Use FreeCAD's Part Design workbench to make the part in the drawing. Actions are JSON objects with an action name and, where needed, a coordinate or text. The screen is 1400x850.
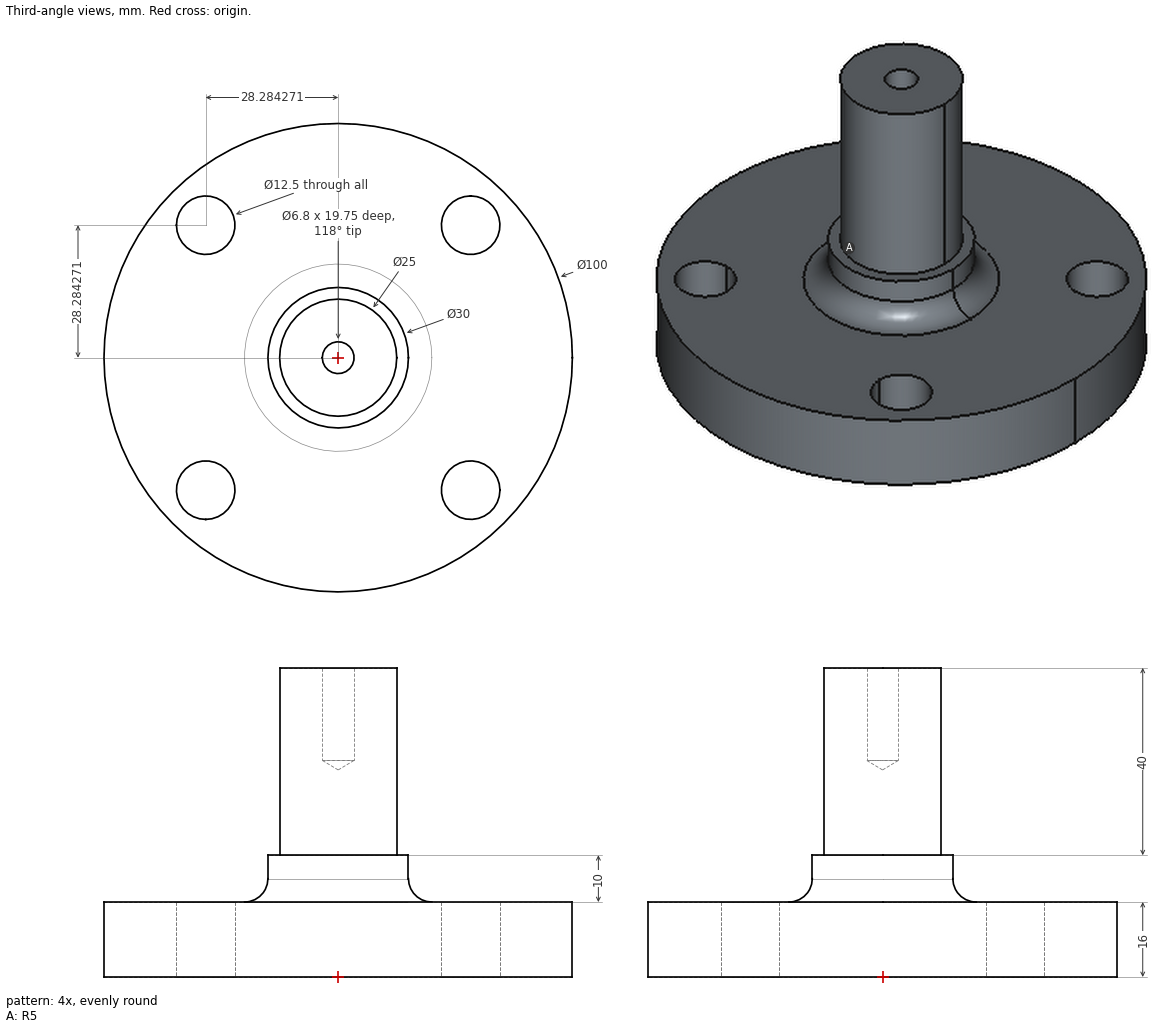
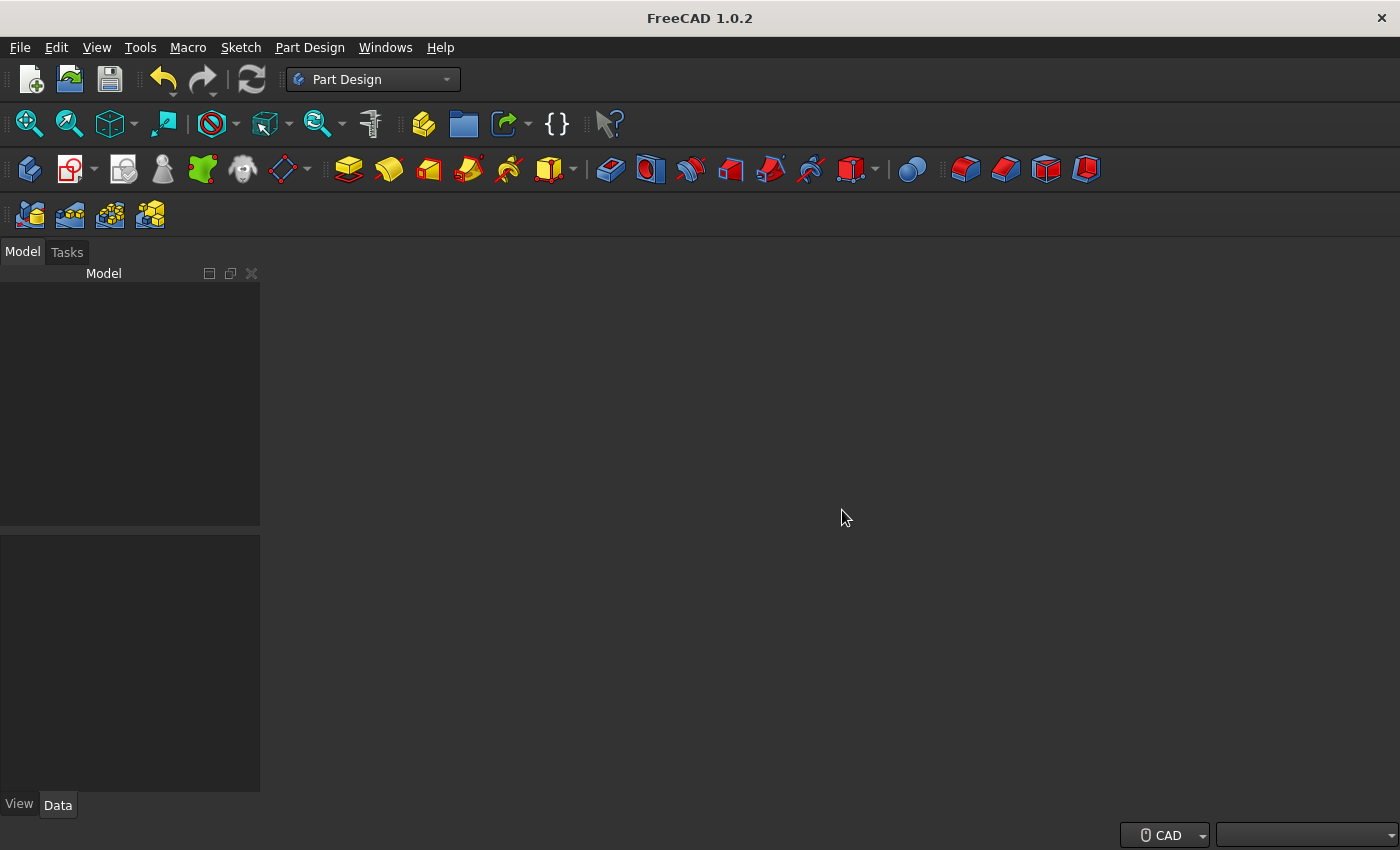
{"action": "key", "text": "ctrl+n"}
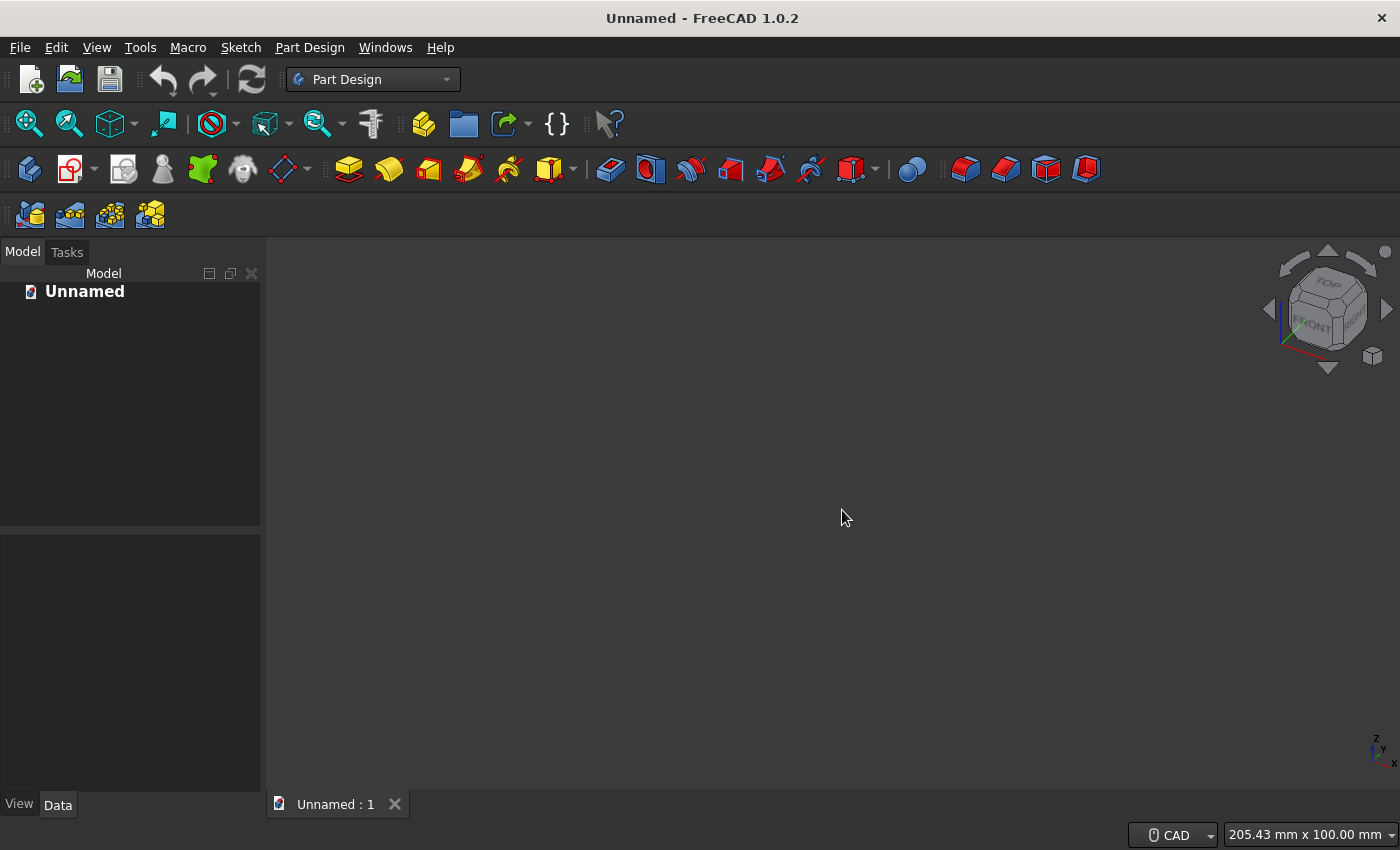
{"action": "left_click", "coordinate": [70, 170]}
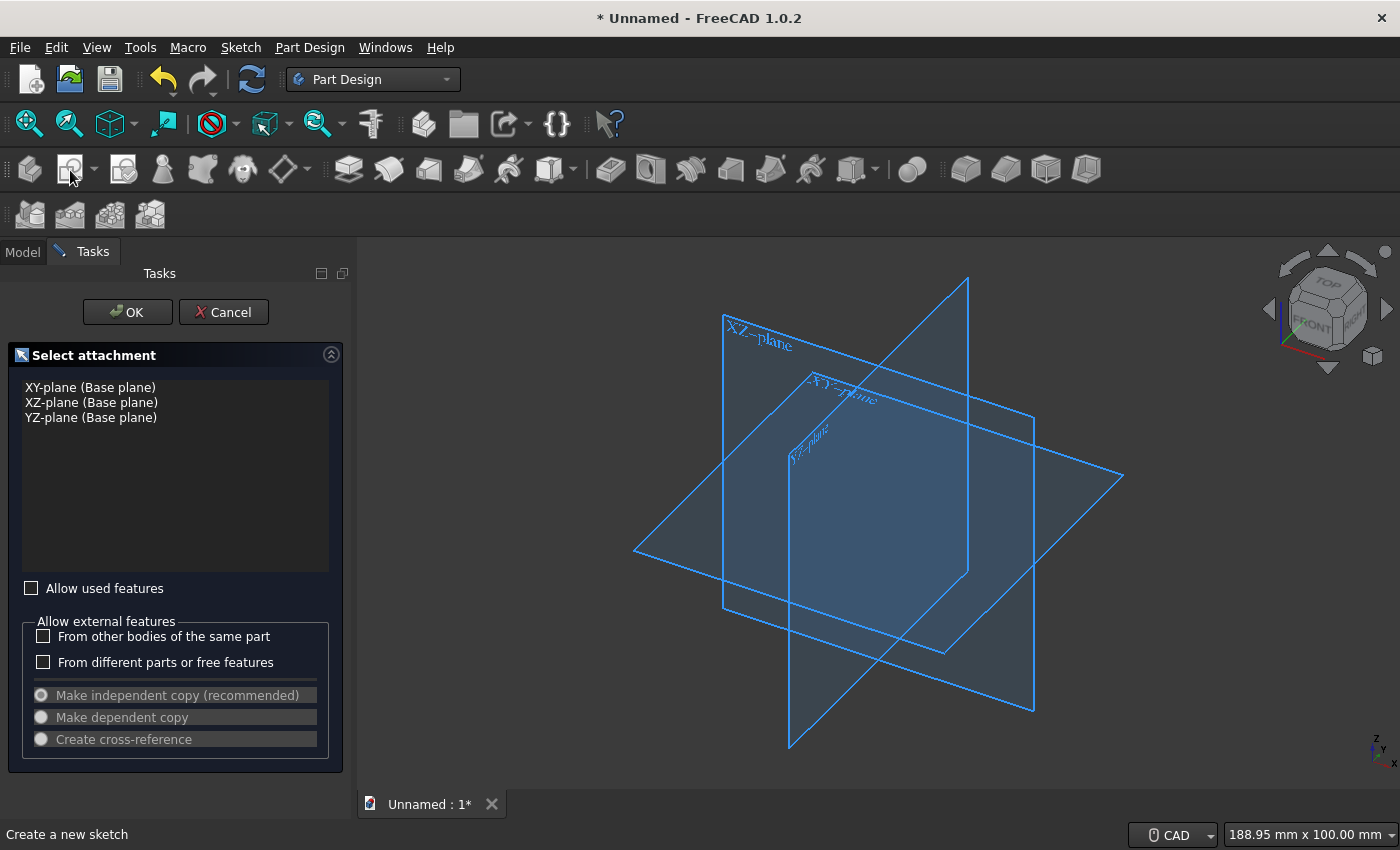
{"action": "left_click", "coordinate": [82, 388]}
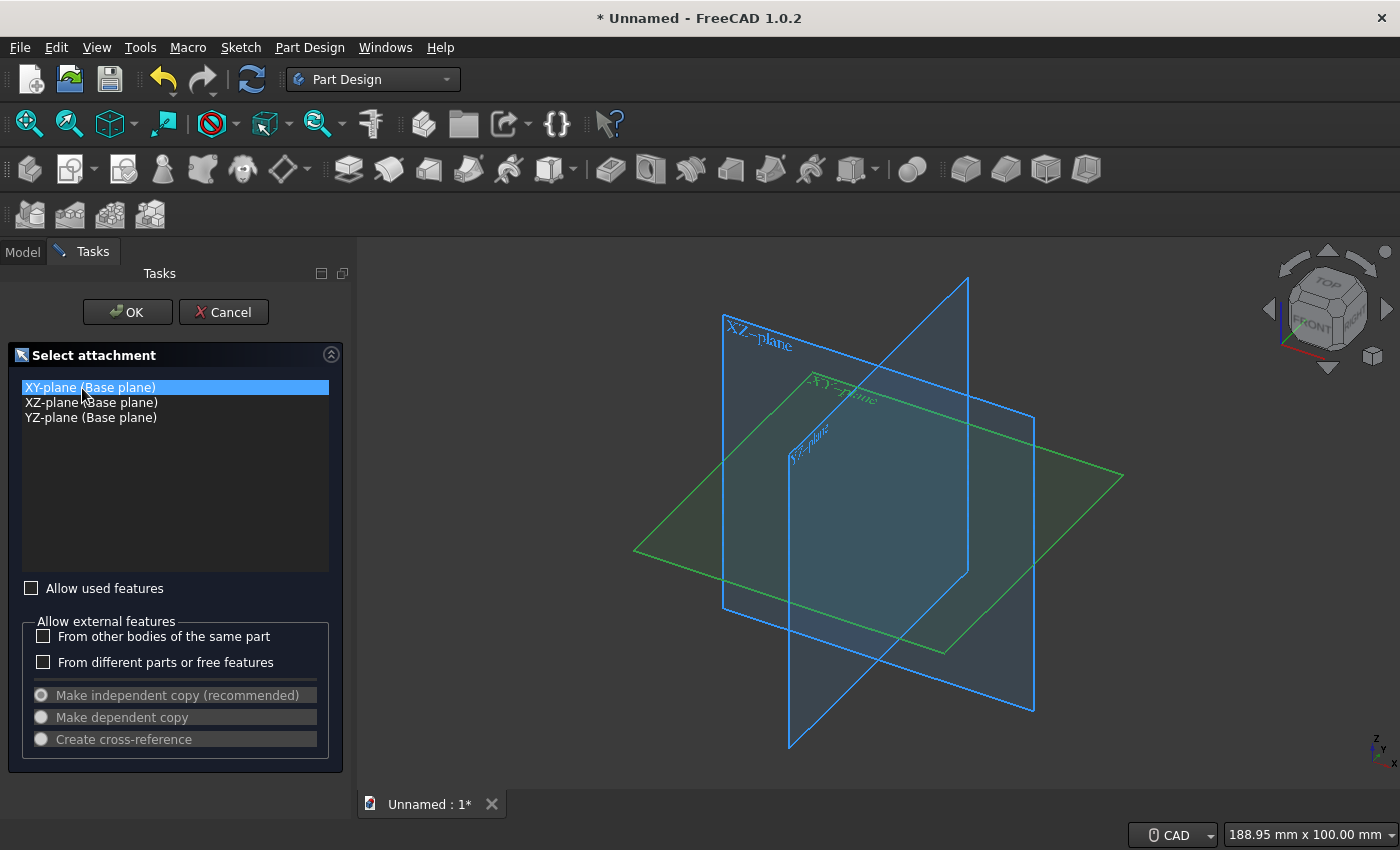
{"action": "left_click", "coordinate": [128, 312]}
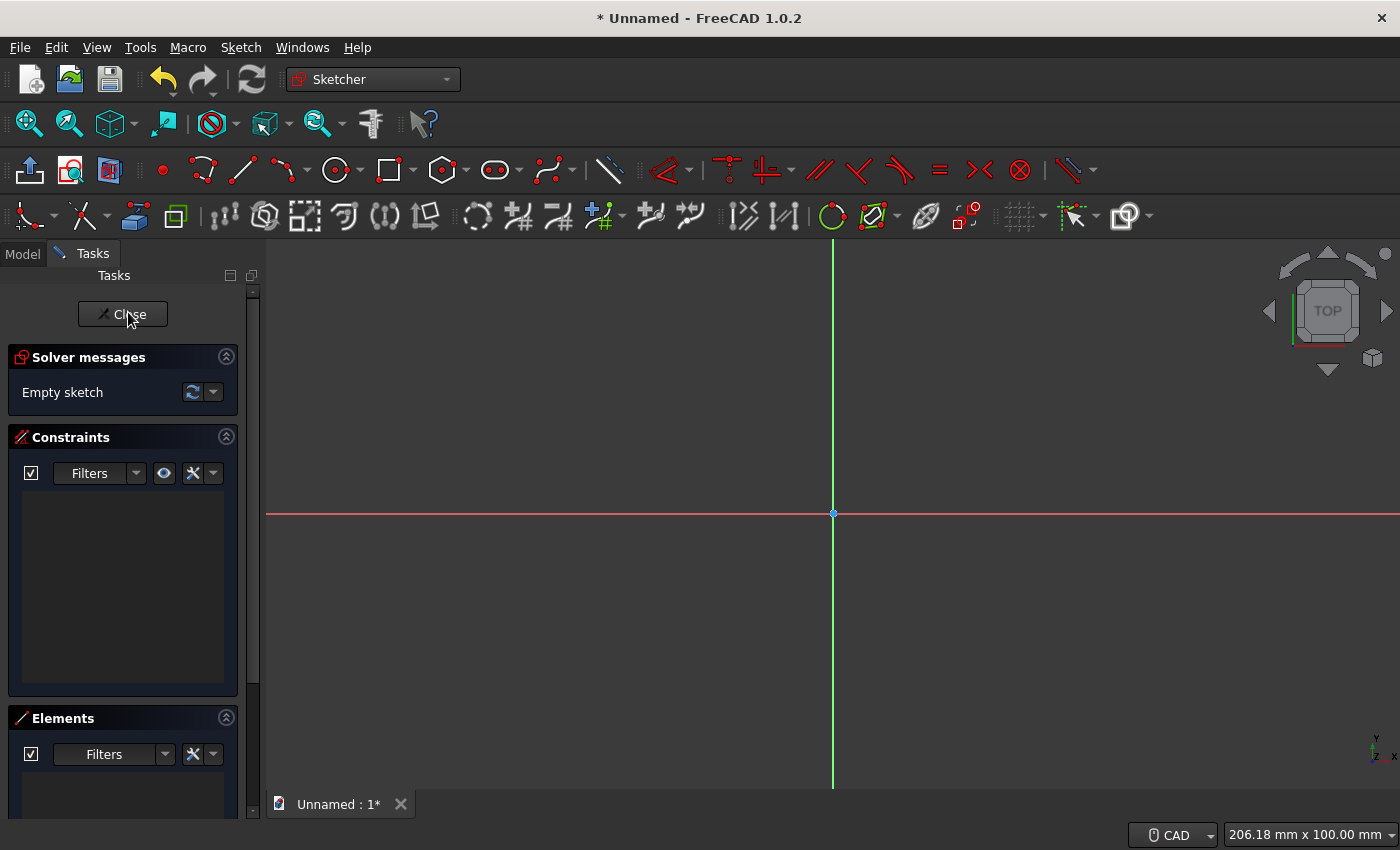
{"action": "scroll", "coordinate": [625, 514], "scroll_direction": "down", "scroll_amount": 2}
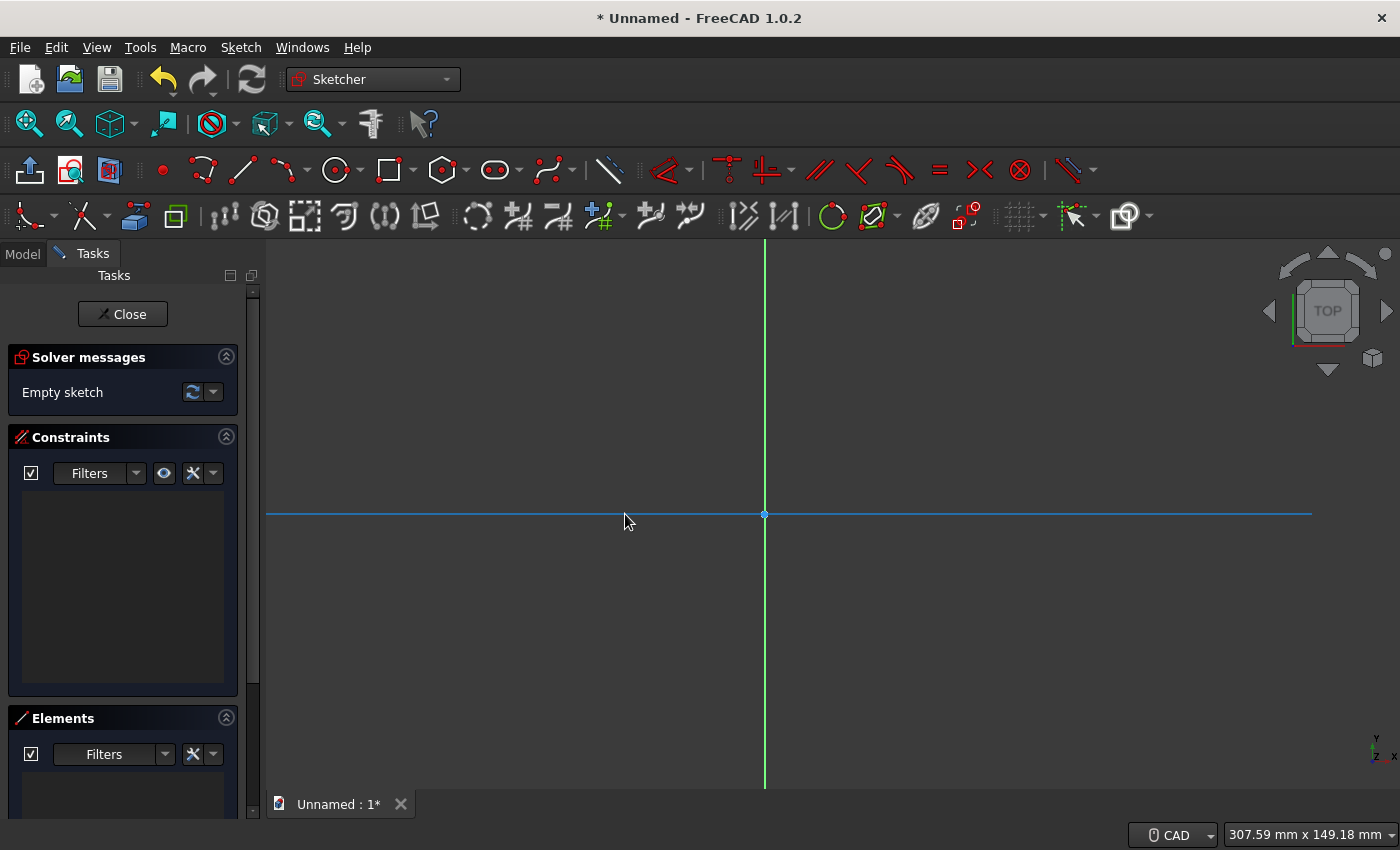
{"action": "key", "text": "g c"}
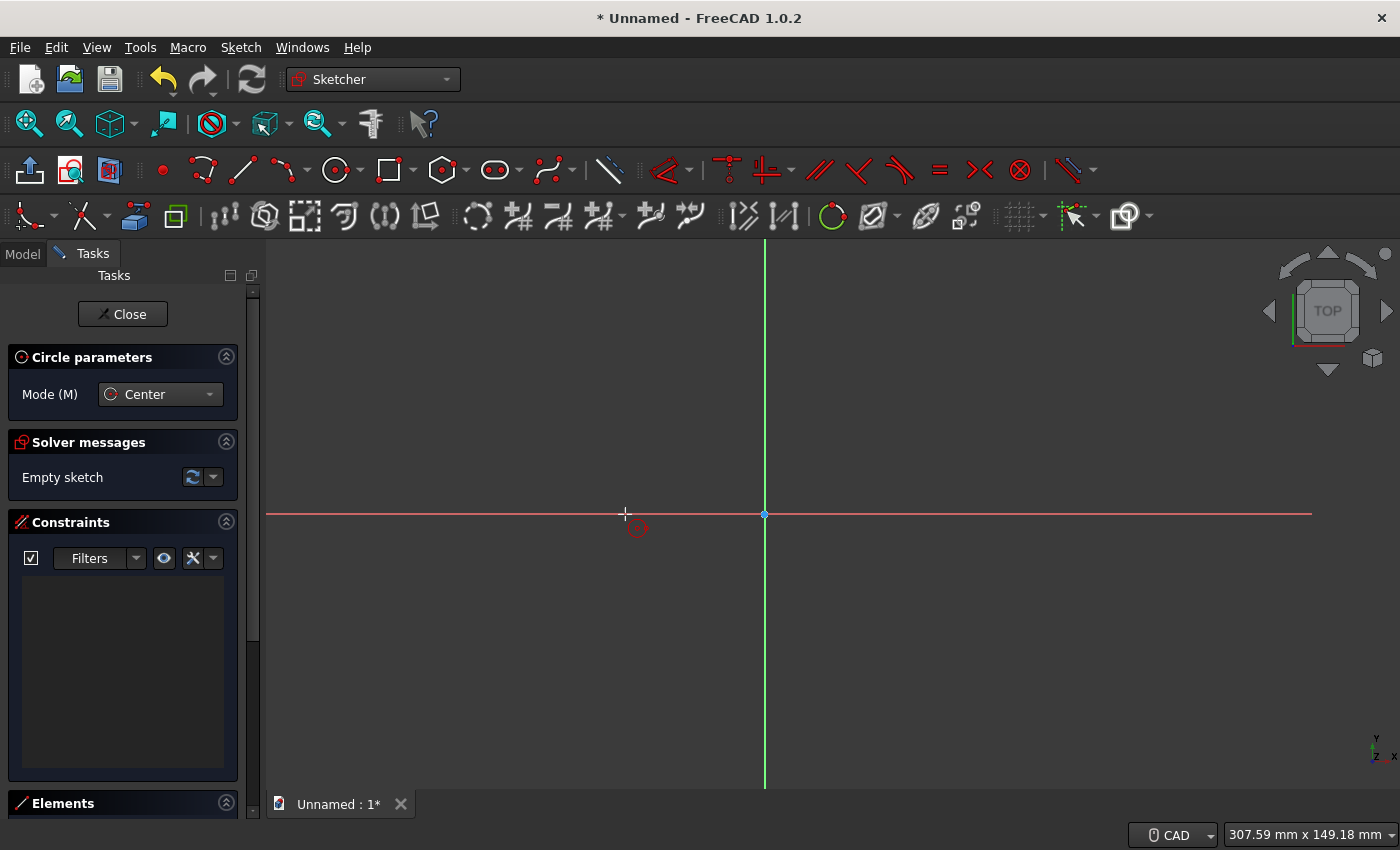
{"action": "left_click", "coordinate": [765, 514]}
{"action": "left_click", "coordinate": [895, 384]}
{"action": "key", "text": "Escape"}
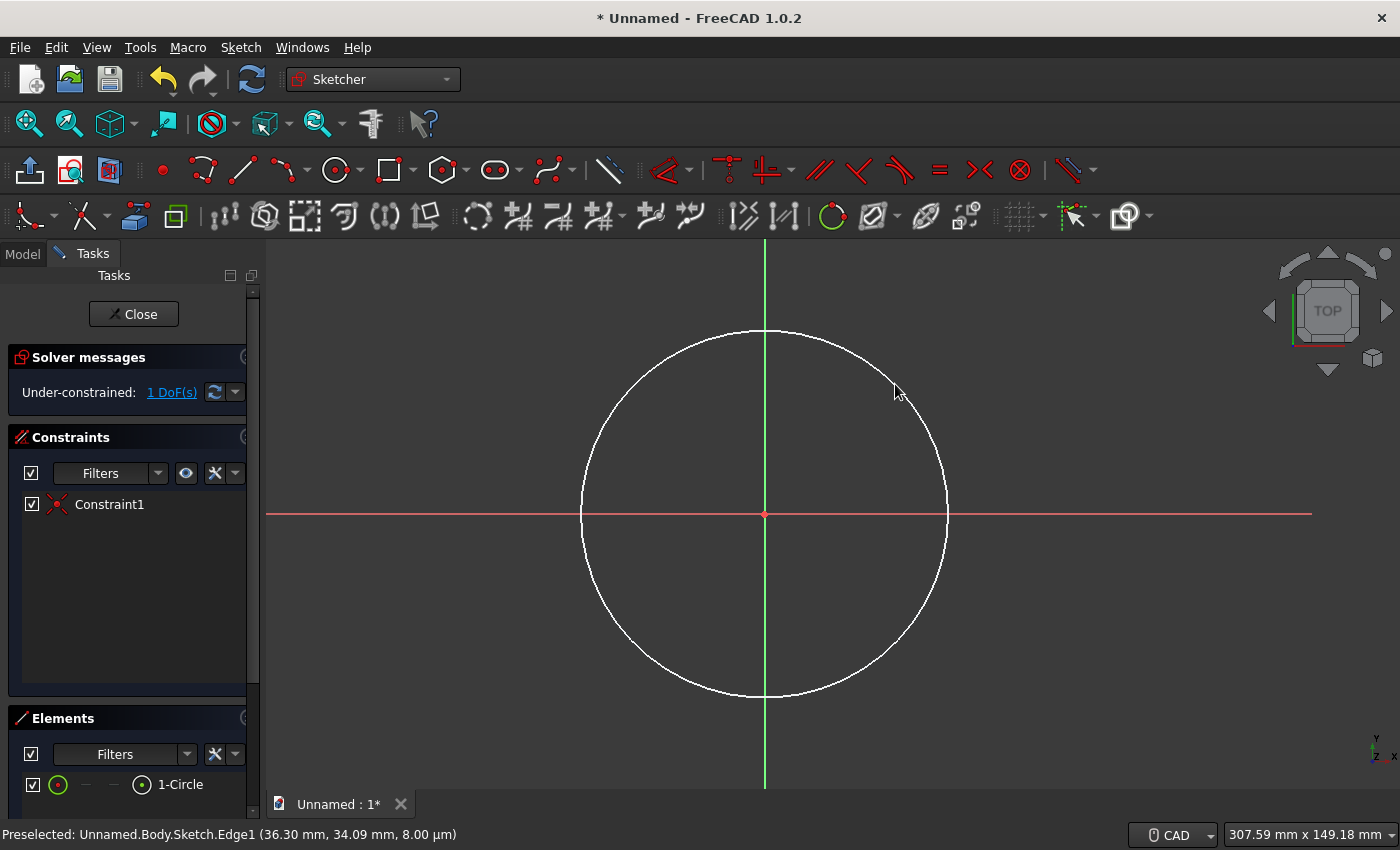
{"action": "key", "text": "d"}